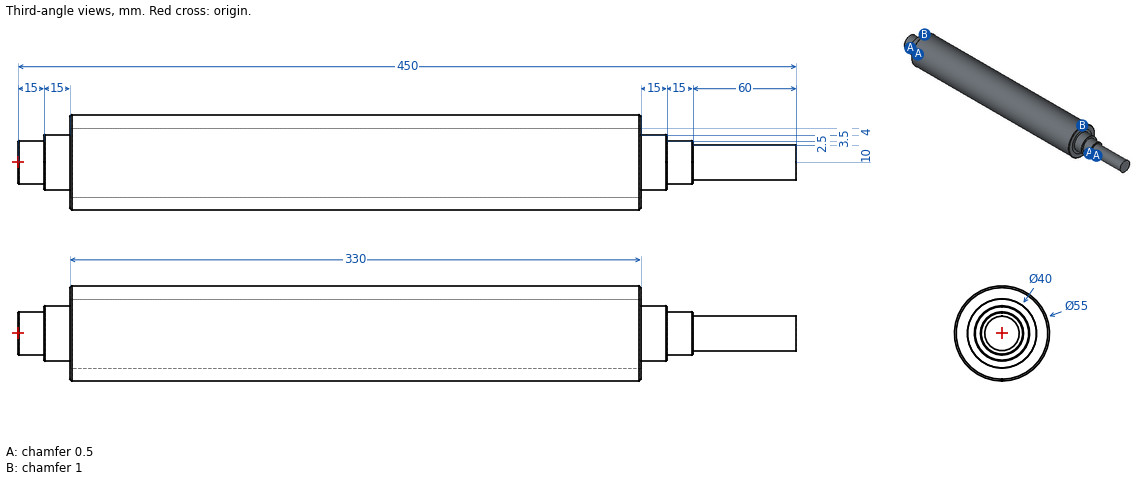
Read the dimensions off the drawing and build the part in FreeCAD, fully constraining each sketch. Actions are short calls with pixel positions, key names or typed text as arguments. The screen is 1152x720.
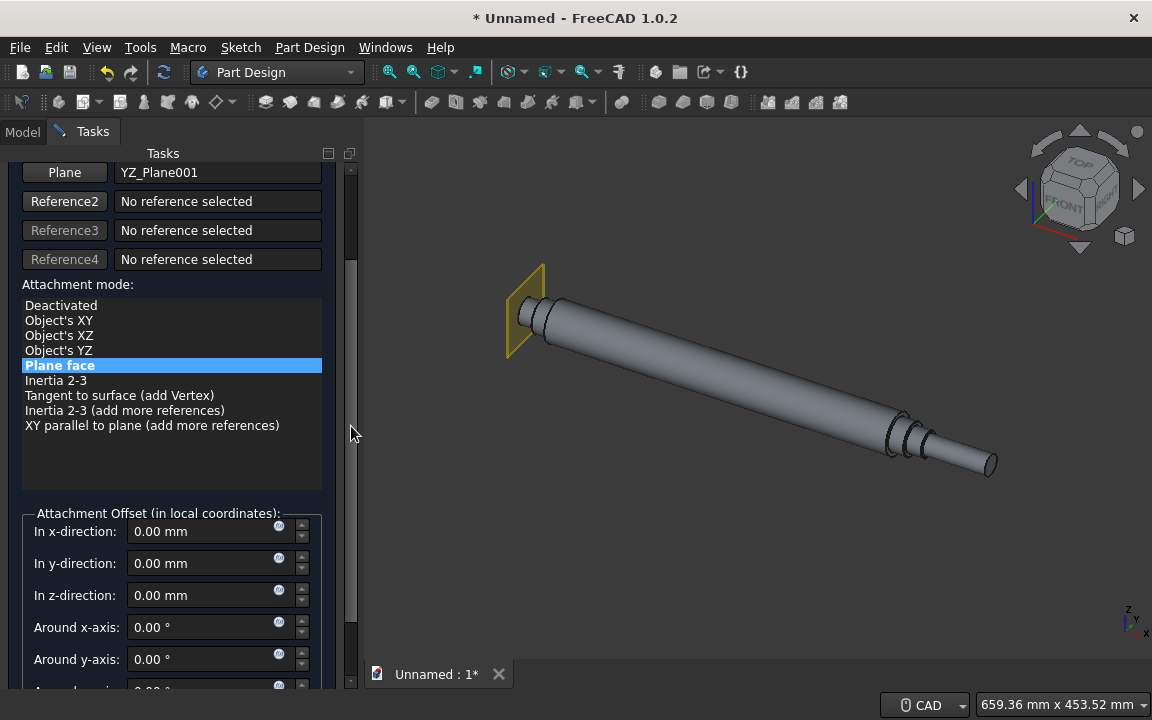
triple_click(210, 595)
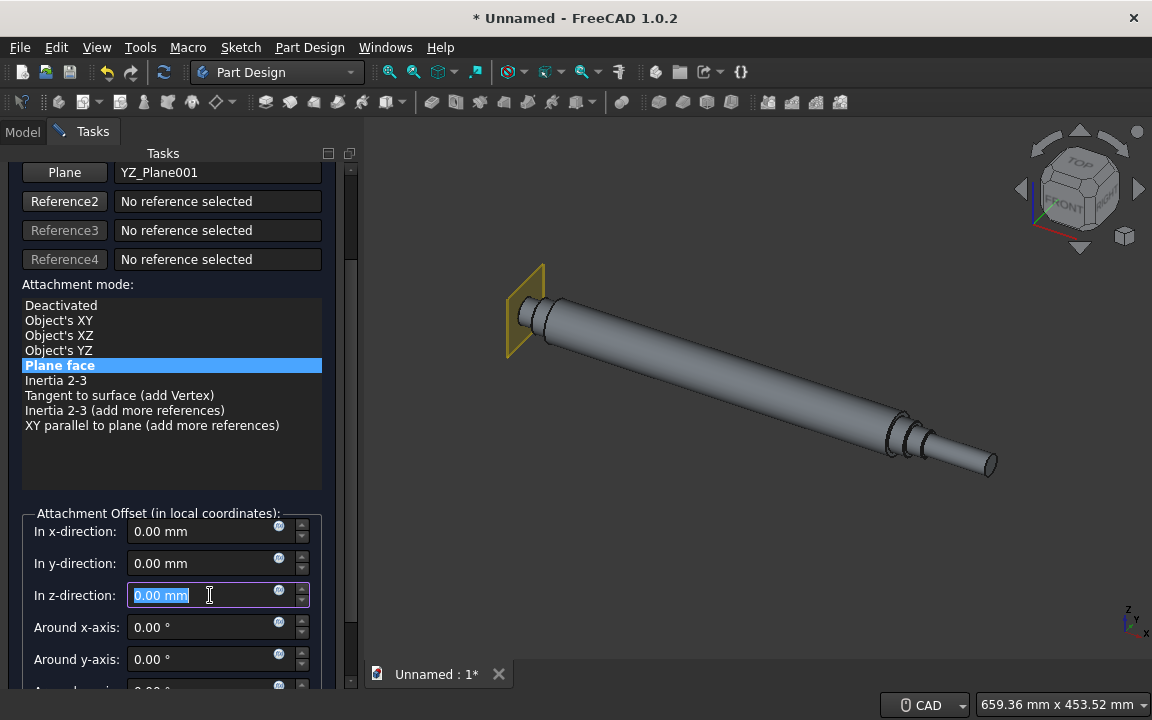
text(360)
key(Tab)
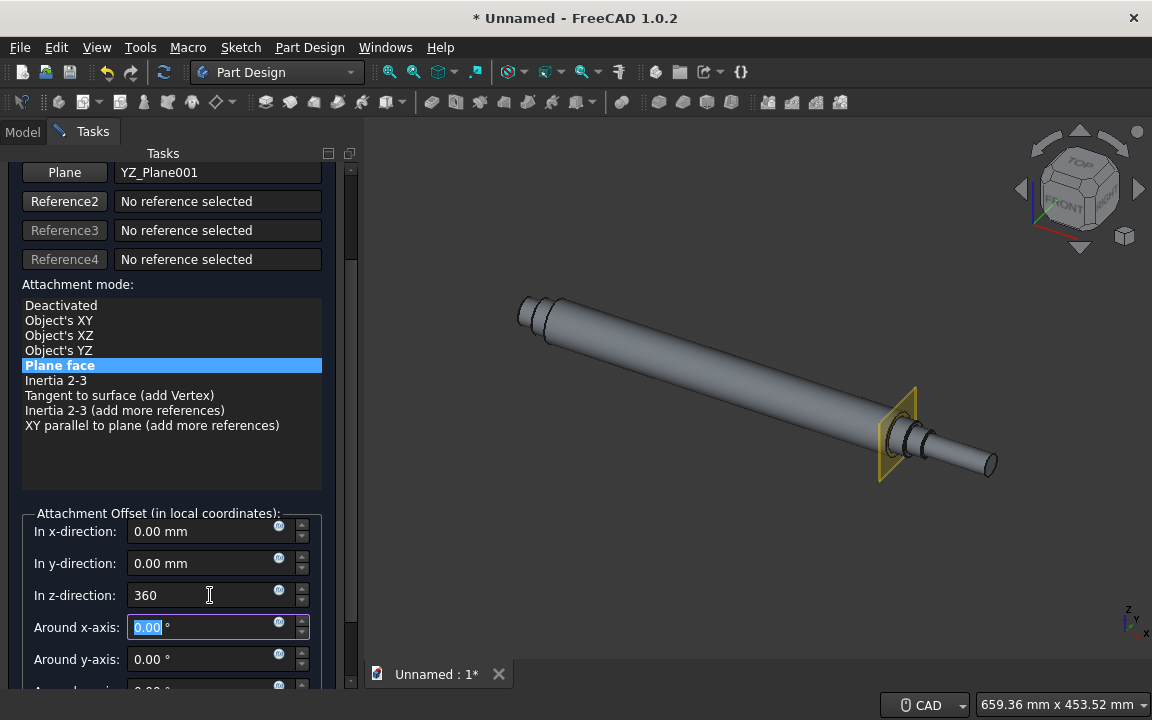
scroll(351, 426, up, 3)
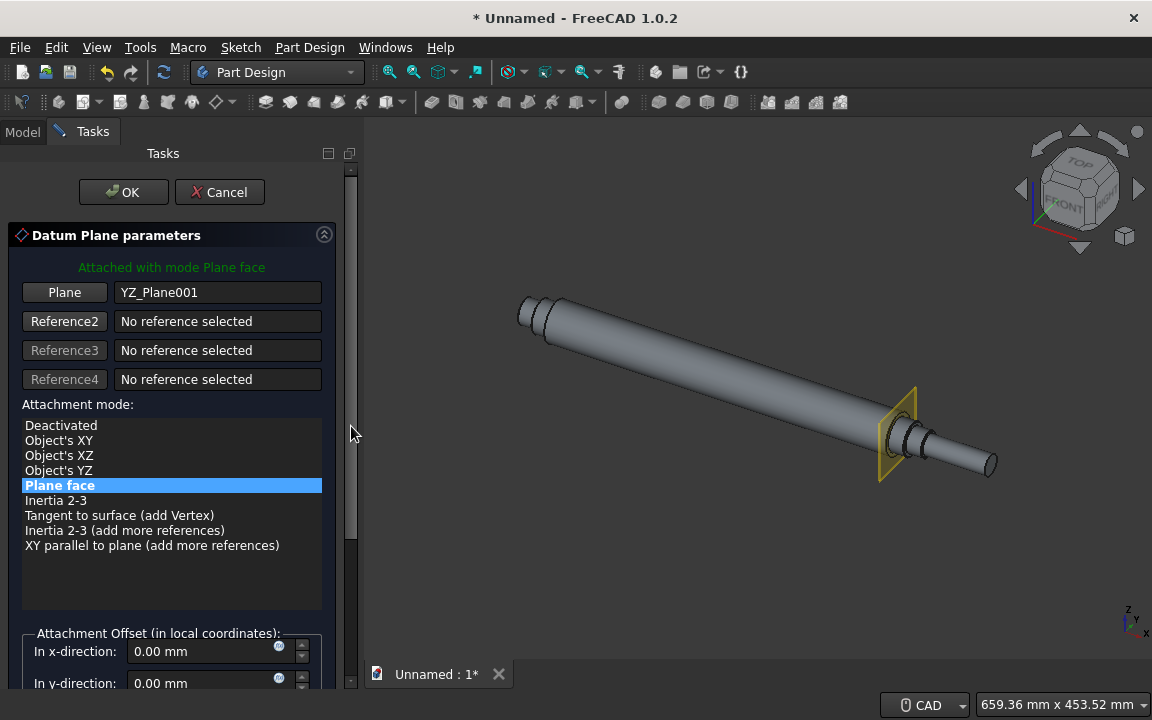
click(124, 192)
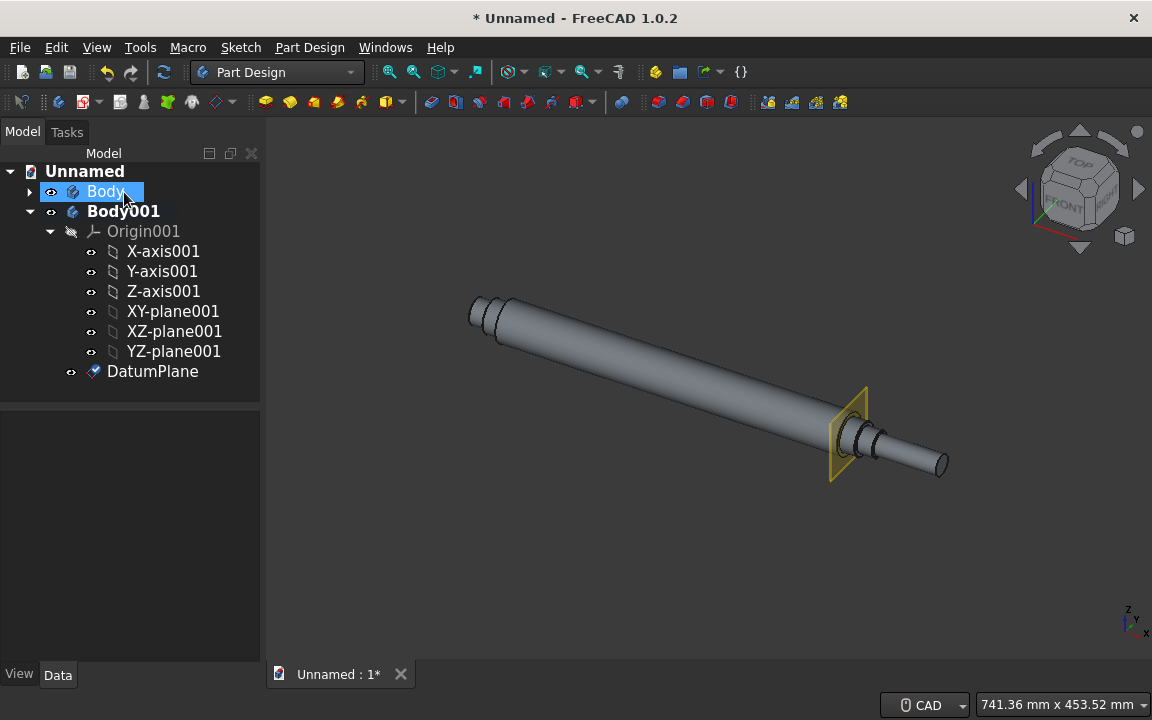
click(116, 372)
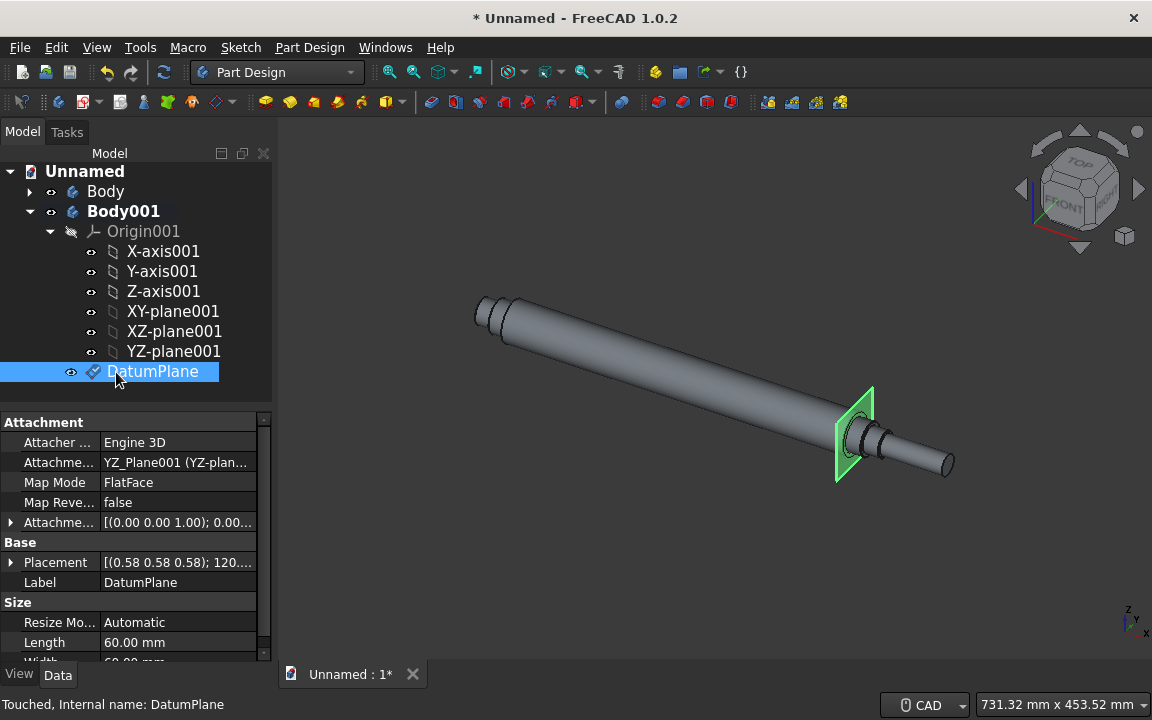
click(84, 102)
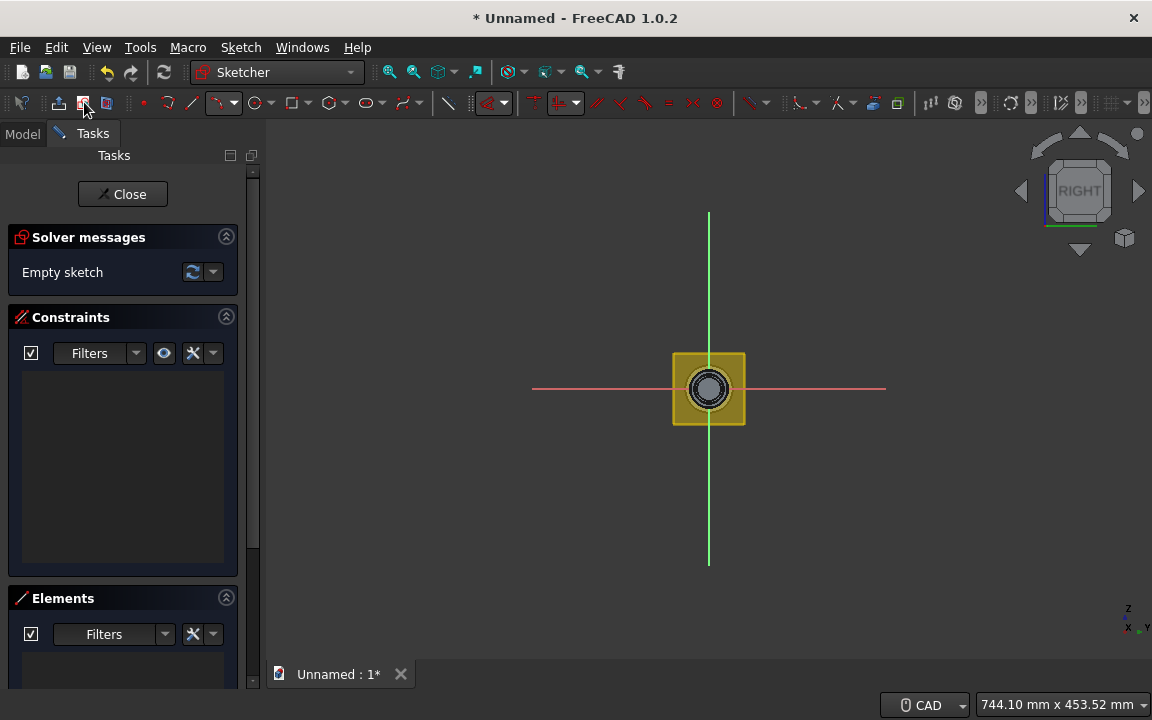
scroll(726, 389, up, 8)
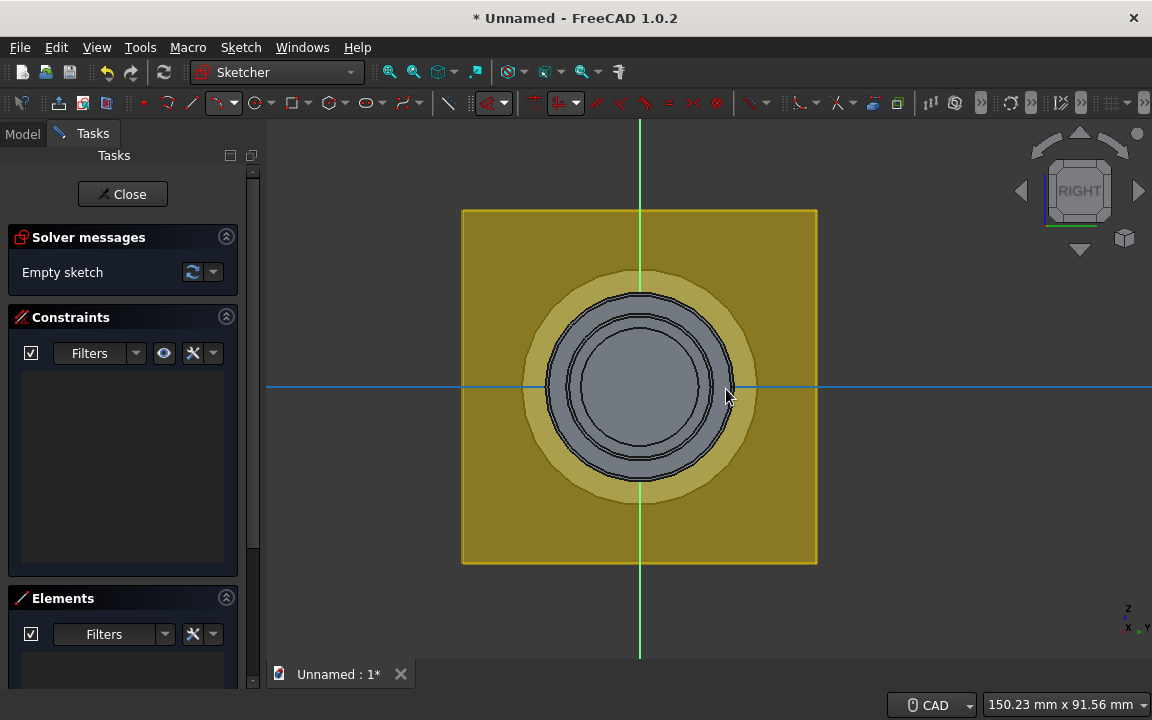
click(256, 104)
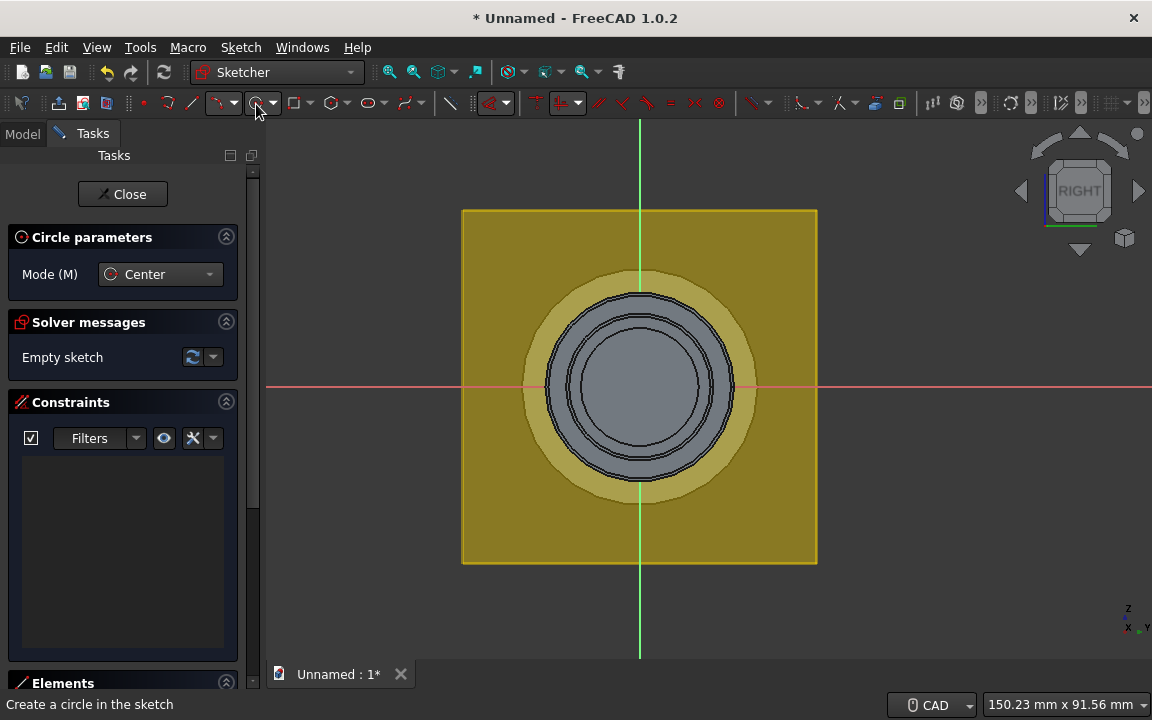
click(640, 387)
click(754, 272)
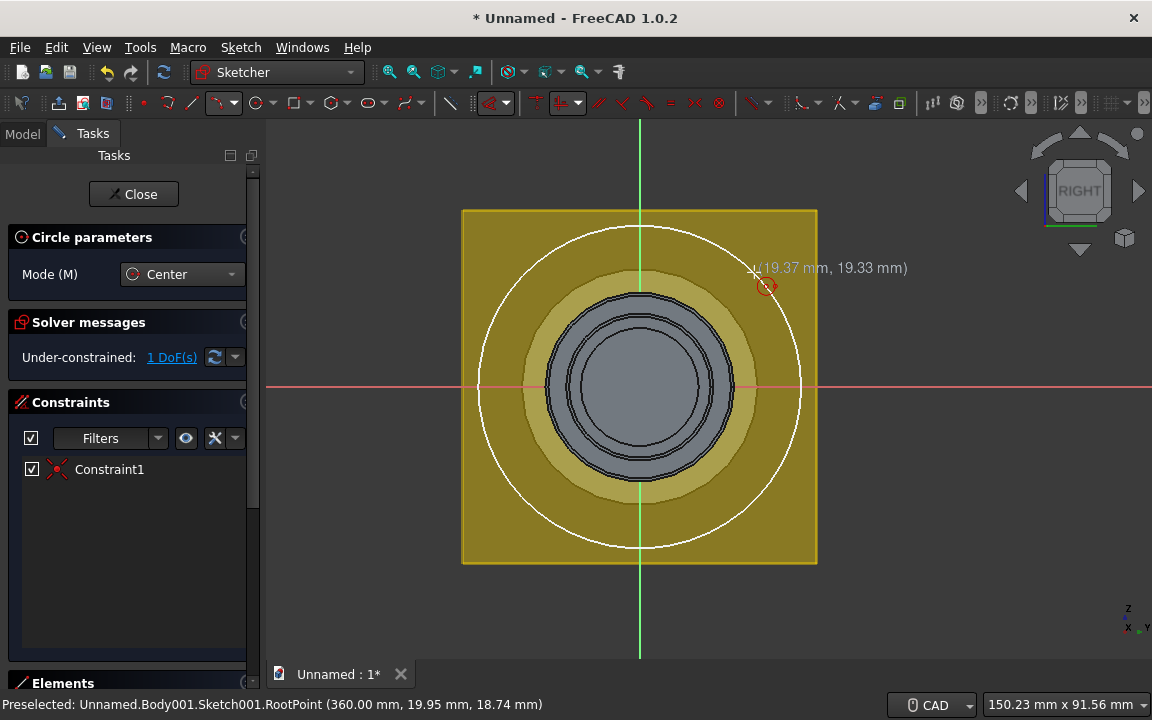
click(640, 387)
click(723, 304)
key(Escape)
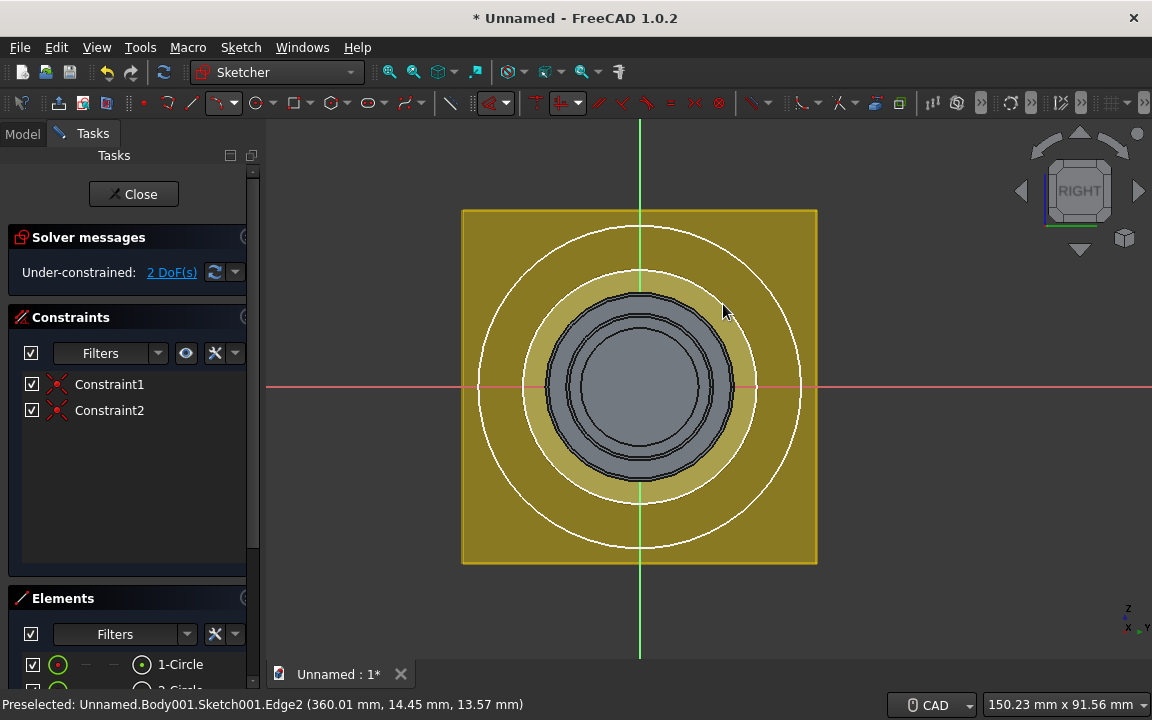
click(490, 104)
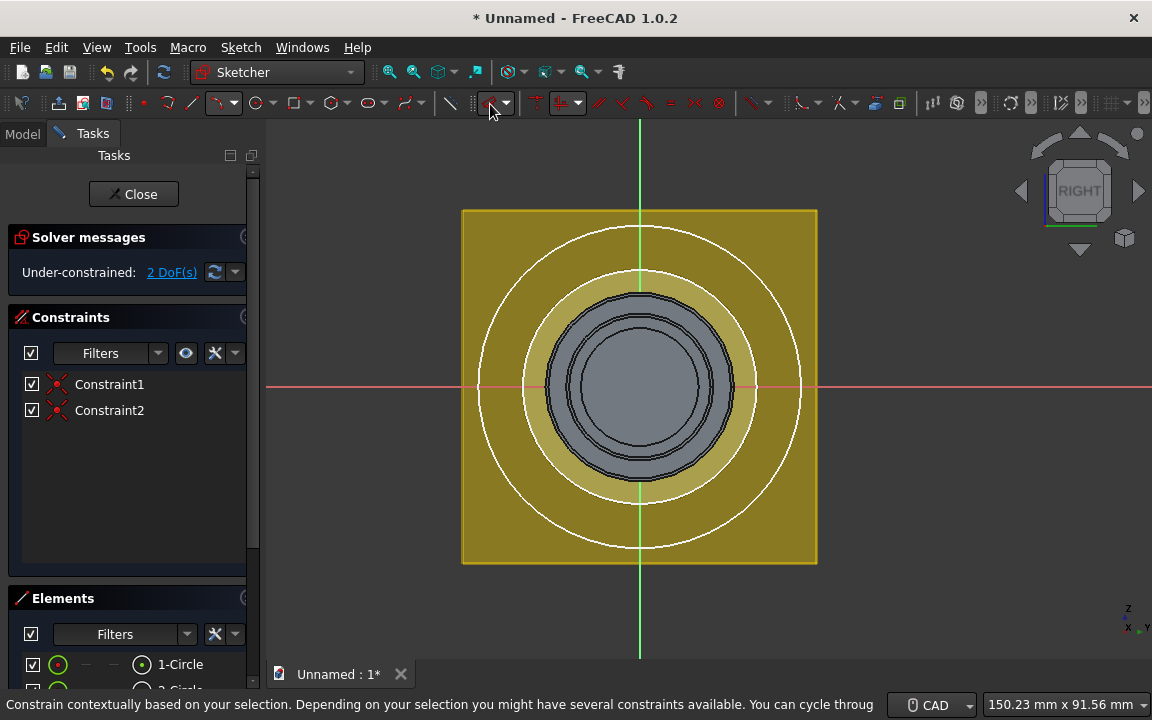
click(754, 273)
click(777, 250)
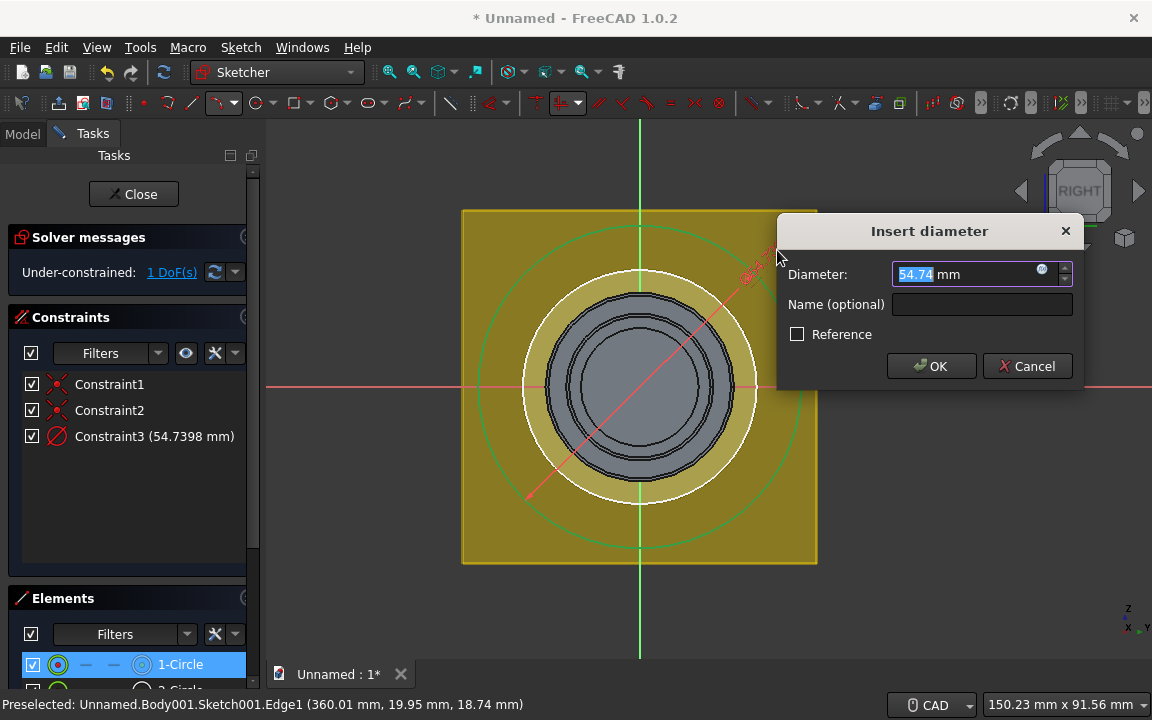
text(55)
key(Return)